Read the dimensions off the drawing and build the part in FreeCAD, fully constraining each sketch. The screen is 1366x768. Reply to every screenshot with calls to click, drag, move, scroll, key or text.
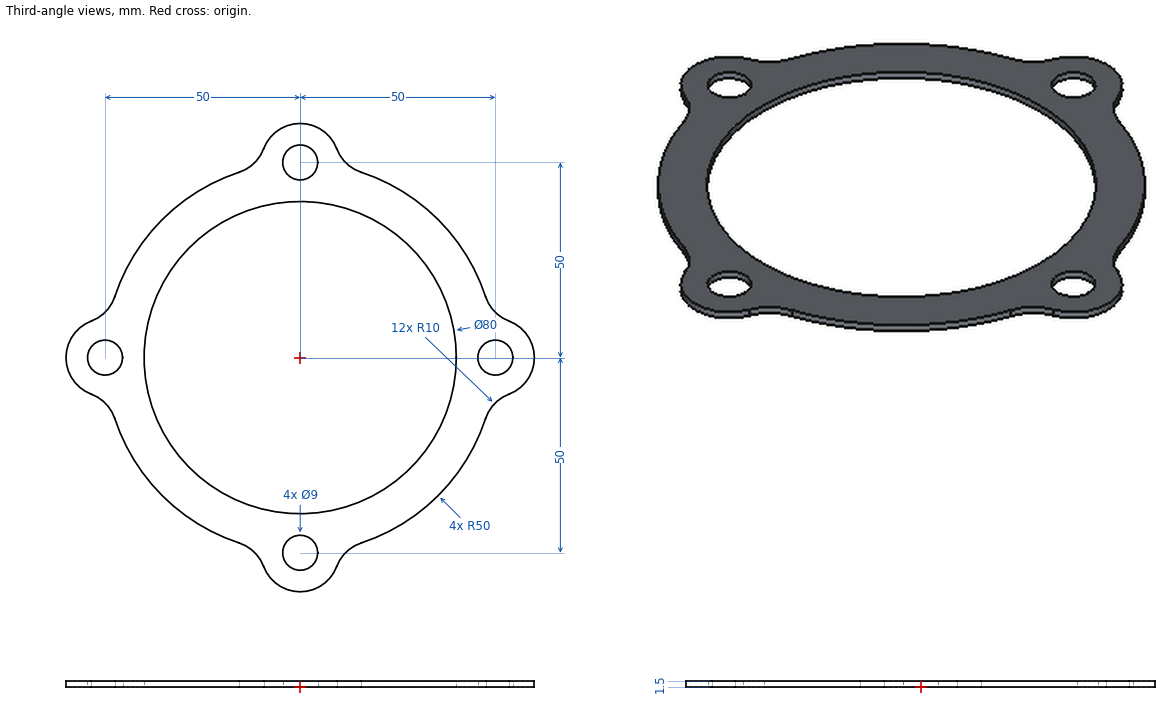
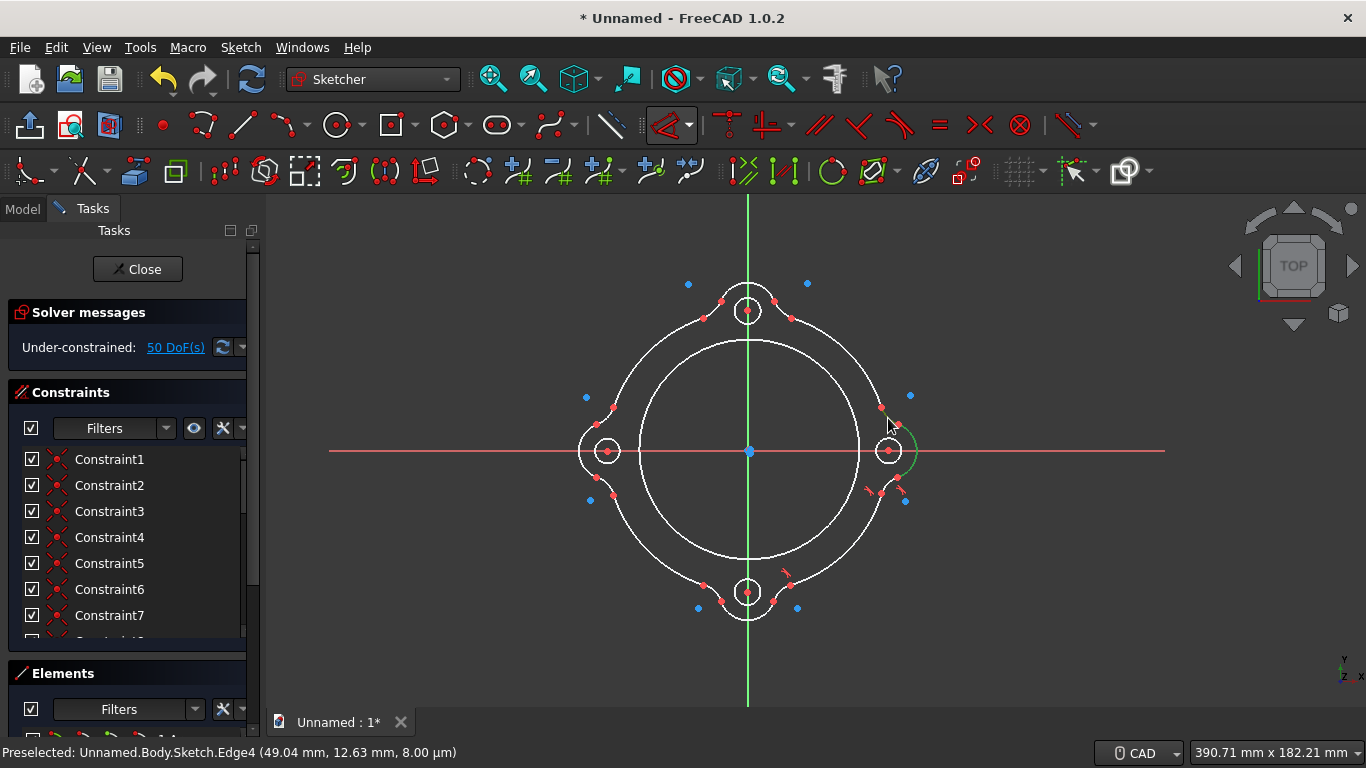
click(900, 126)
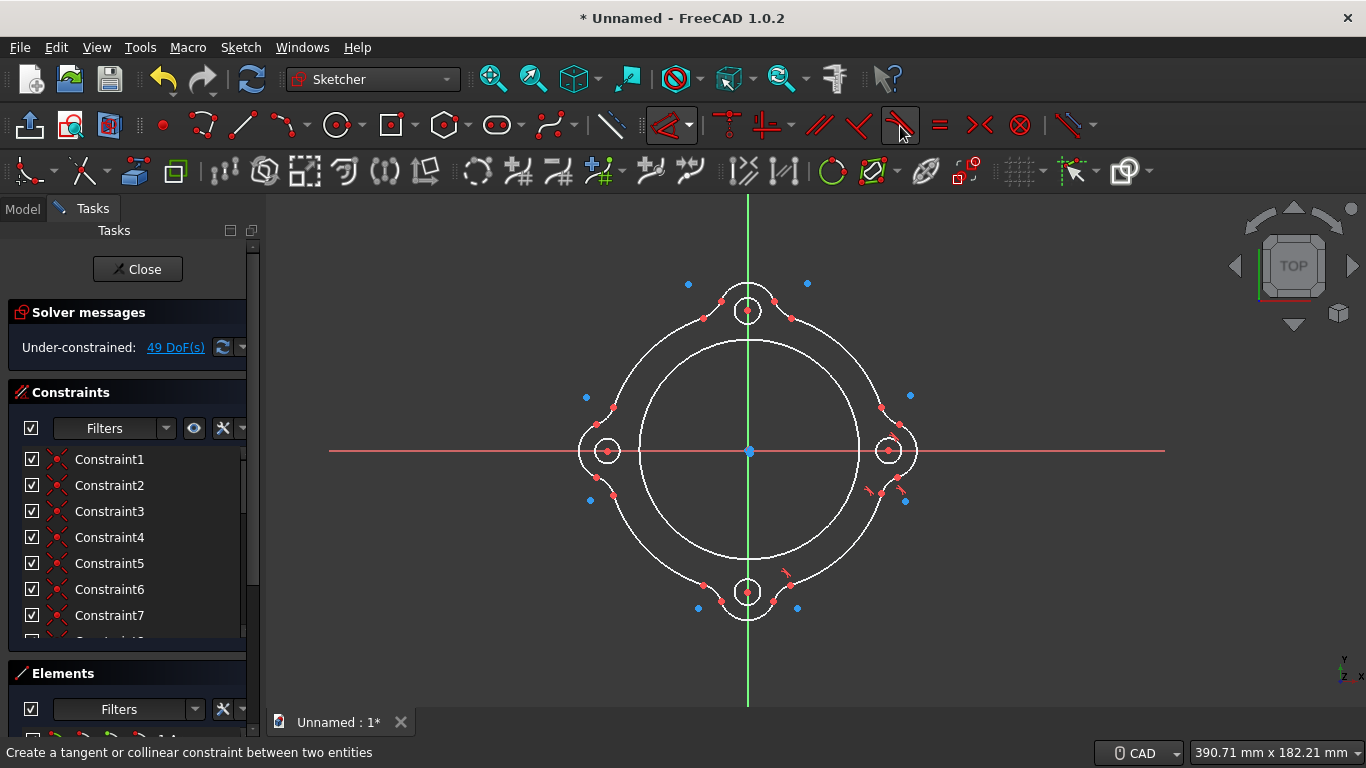
click(889, 418)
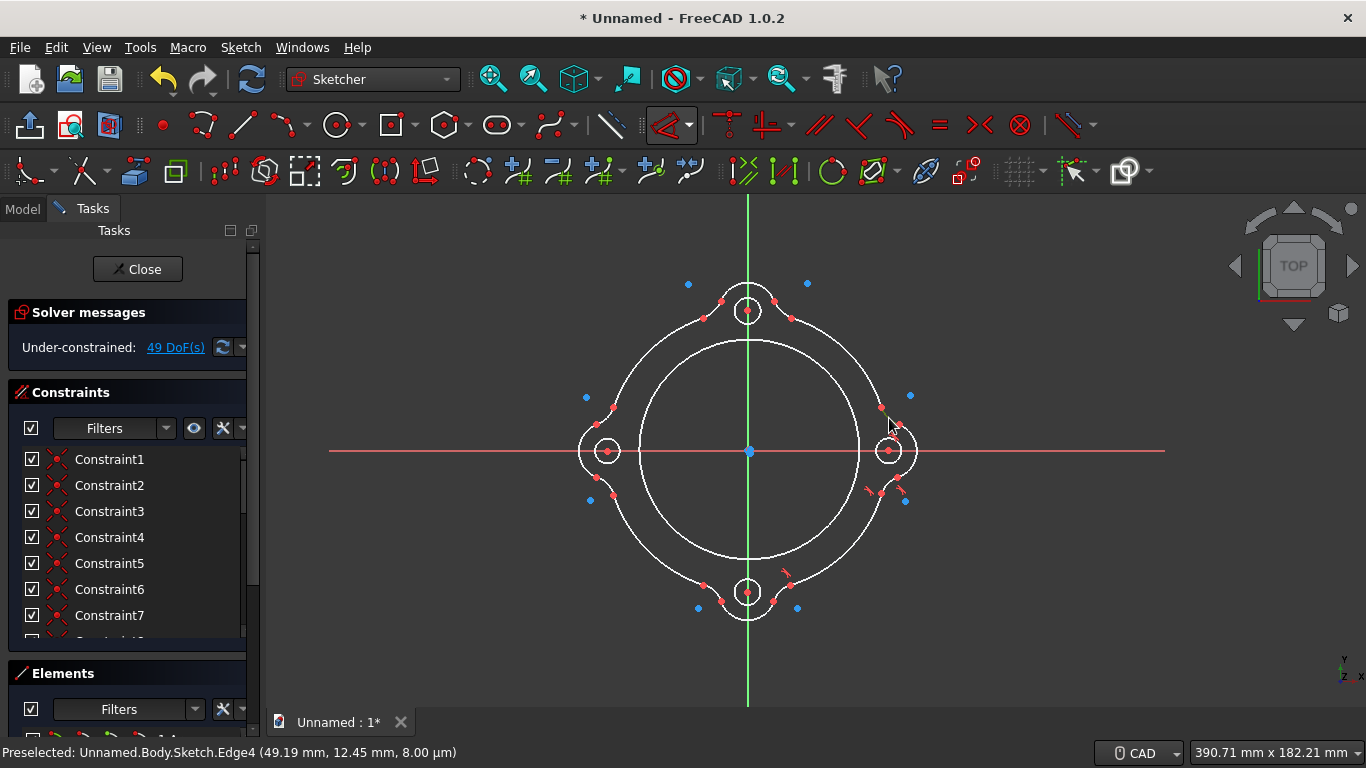
click(865, 372)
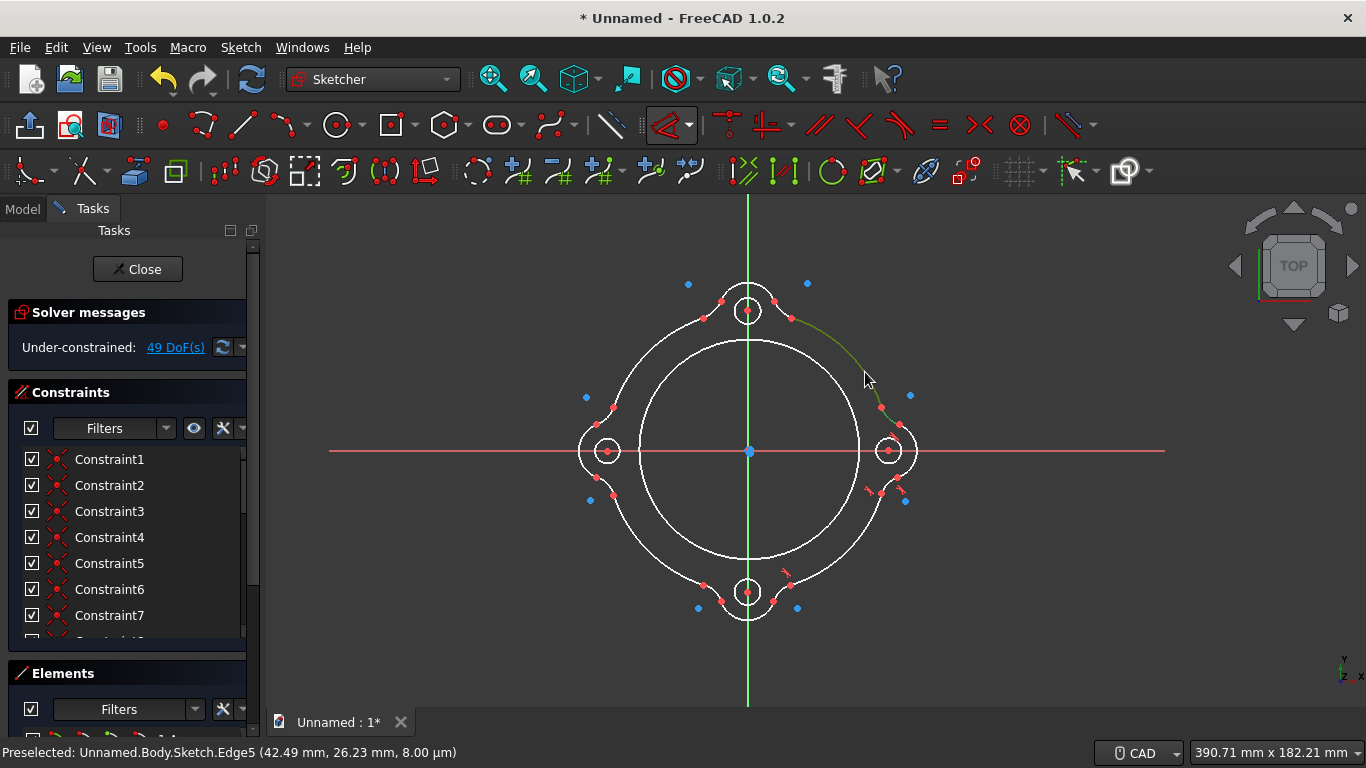
click(900, 126)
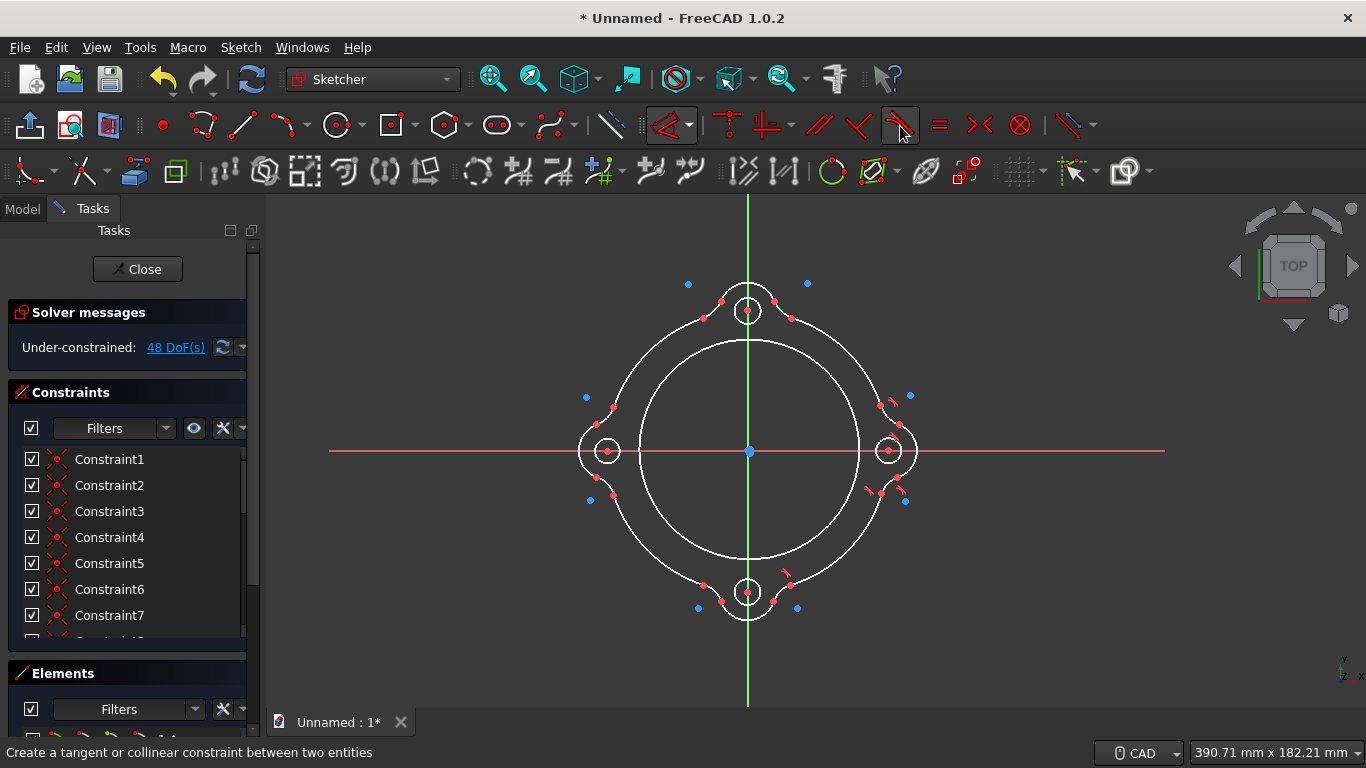
click(864, 371)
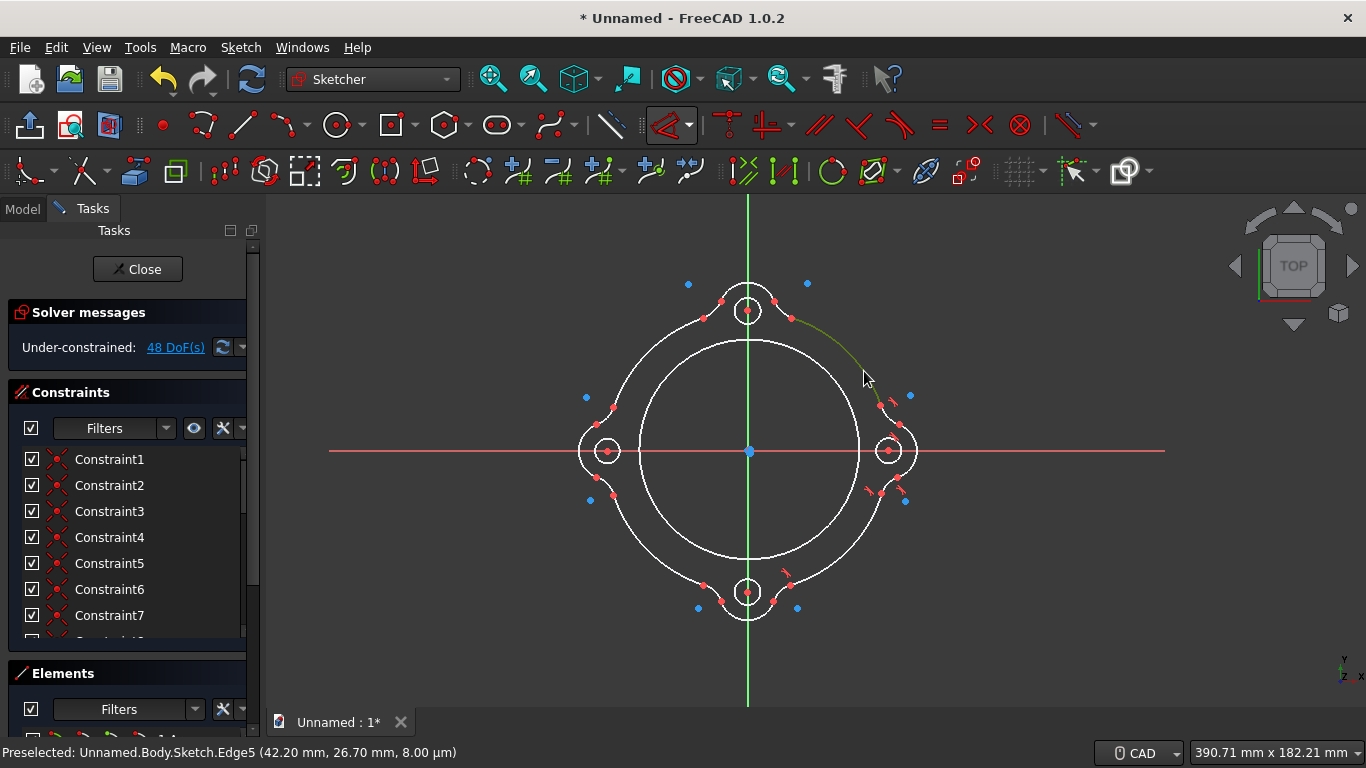
click(782, 311)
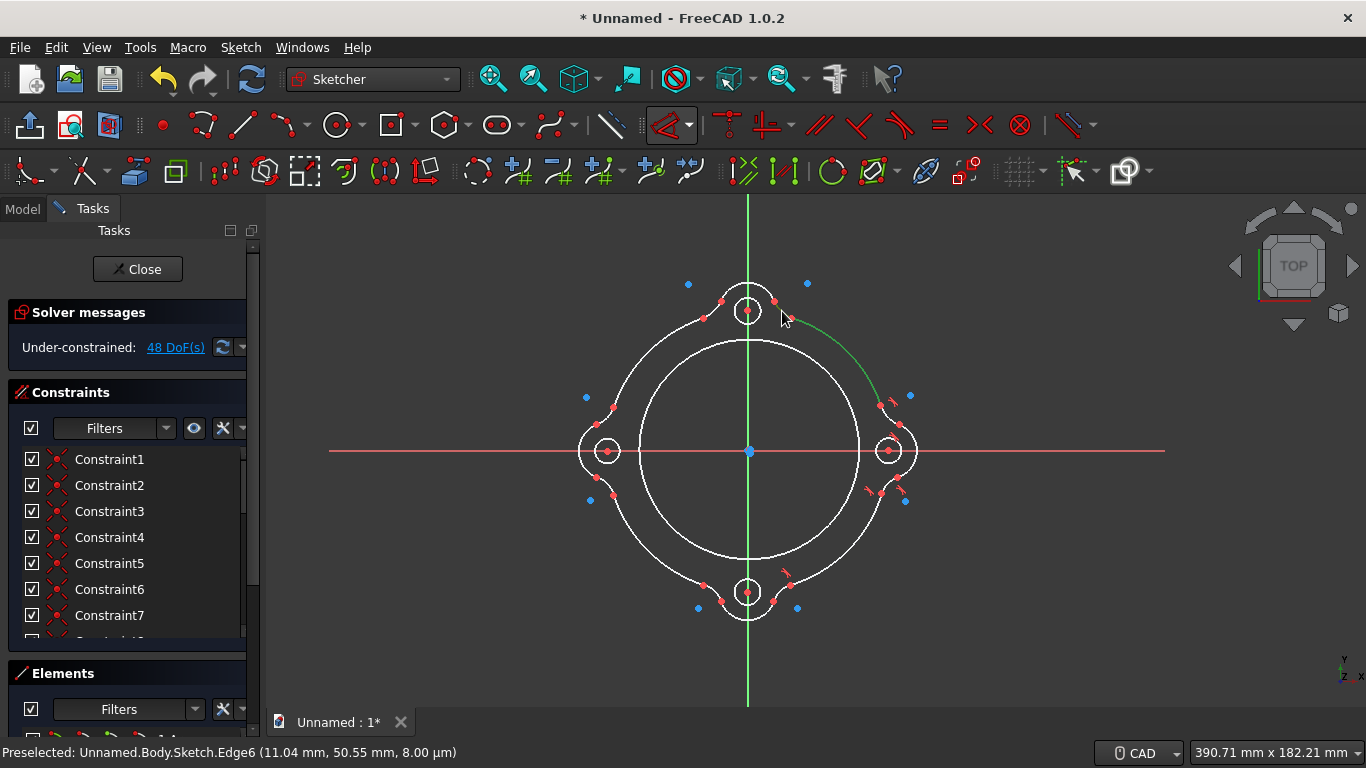
click(900, 126)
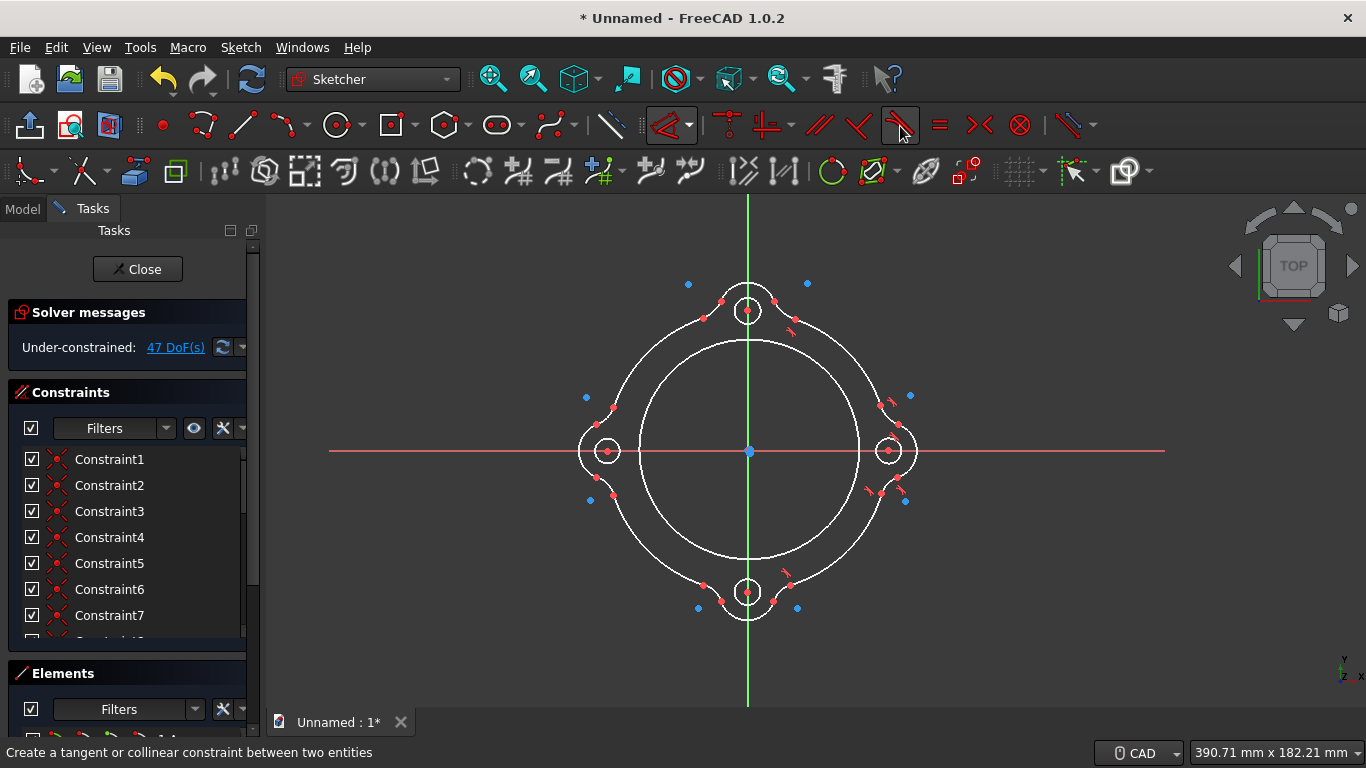
click(783, 312)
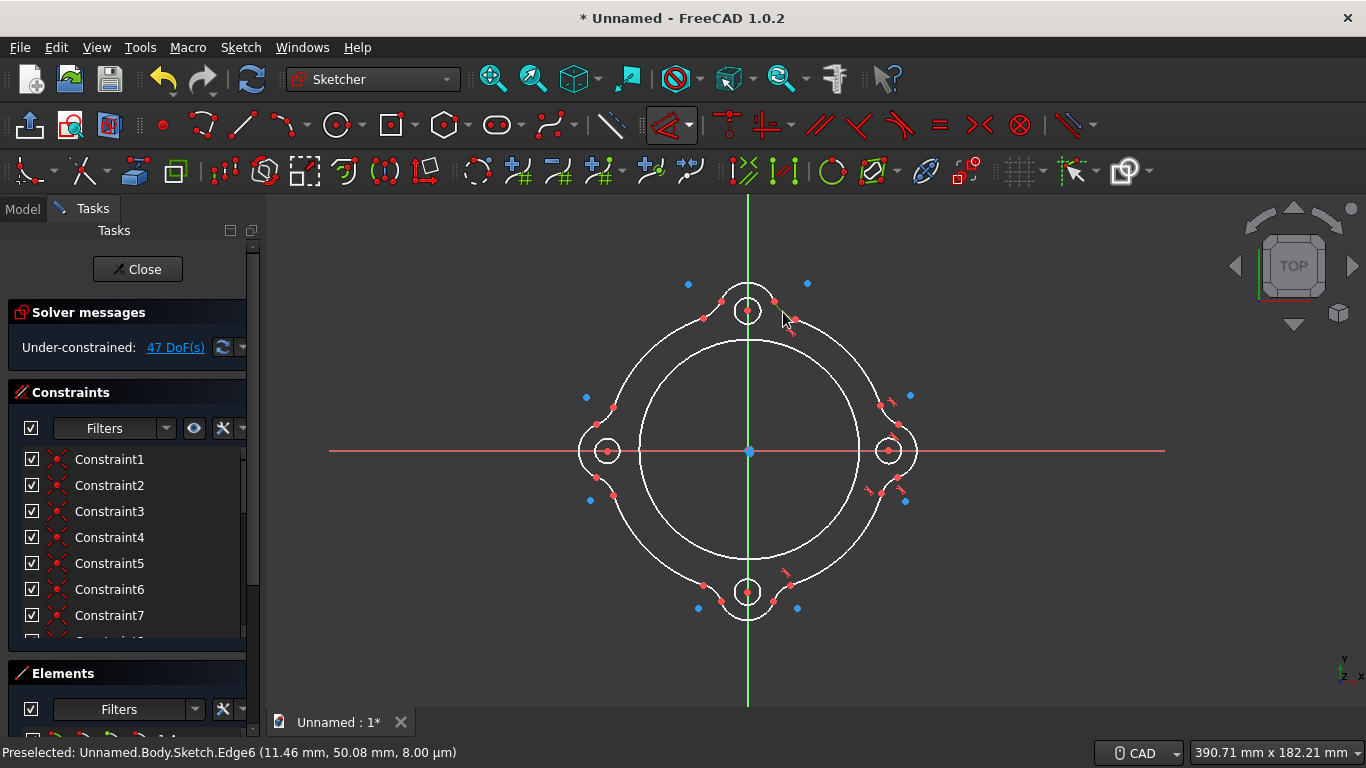
click(761, 286)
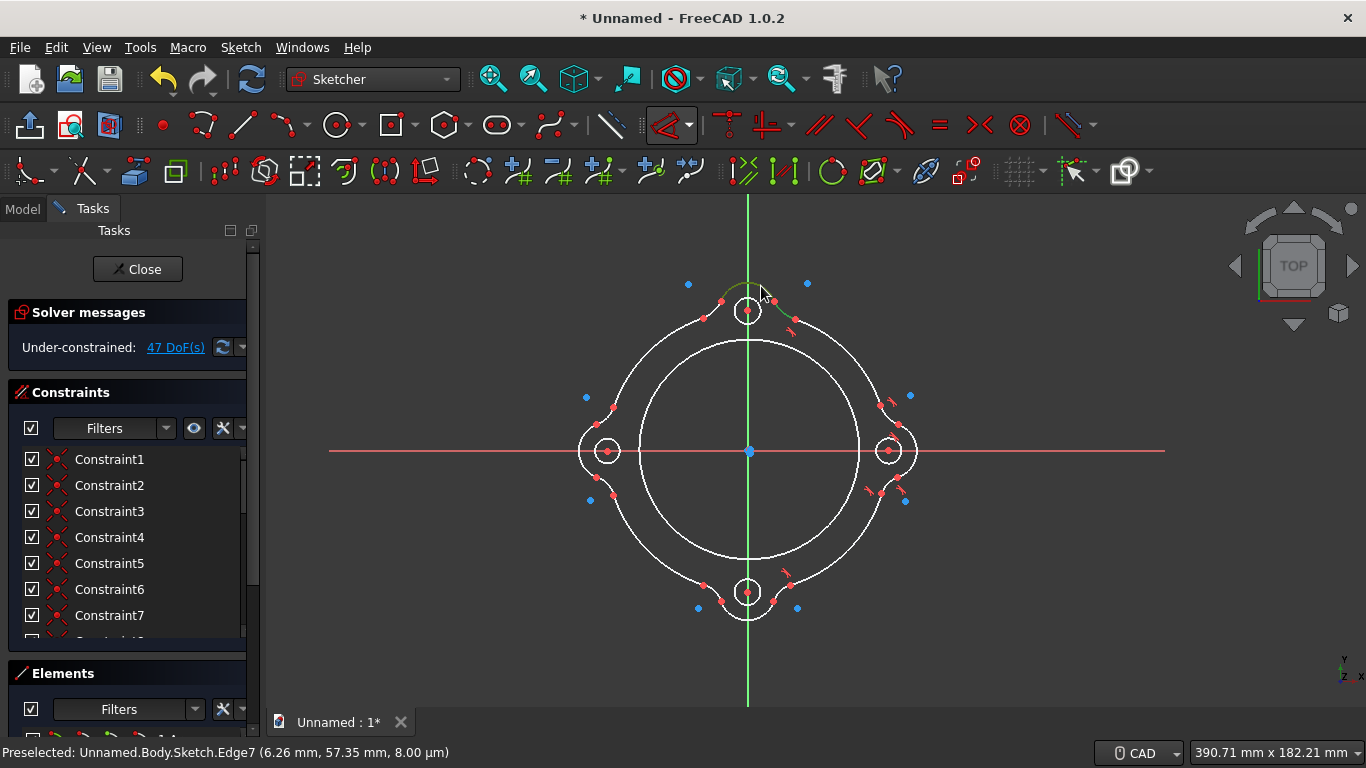
click(900, 126)